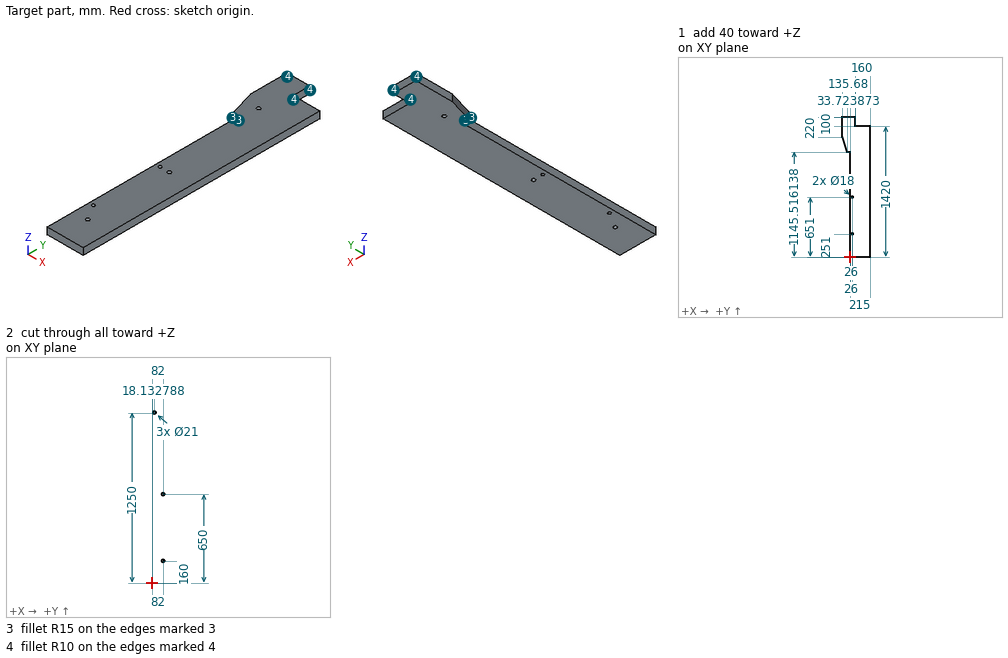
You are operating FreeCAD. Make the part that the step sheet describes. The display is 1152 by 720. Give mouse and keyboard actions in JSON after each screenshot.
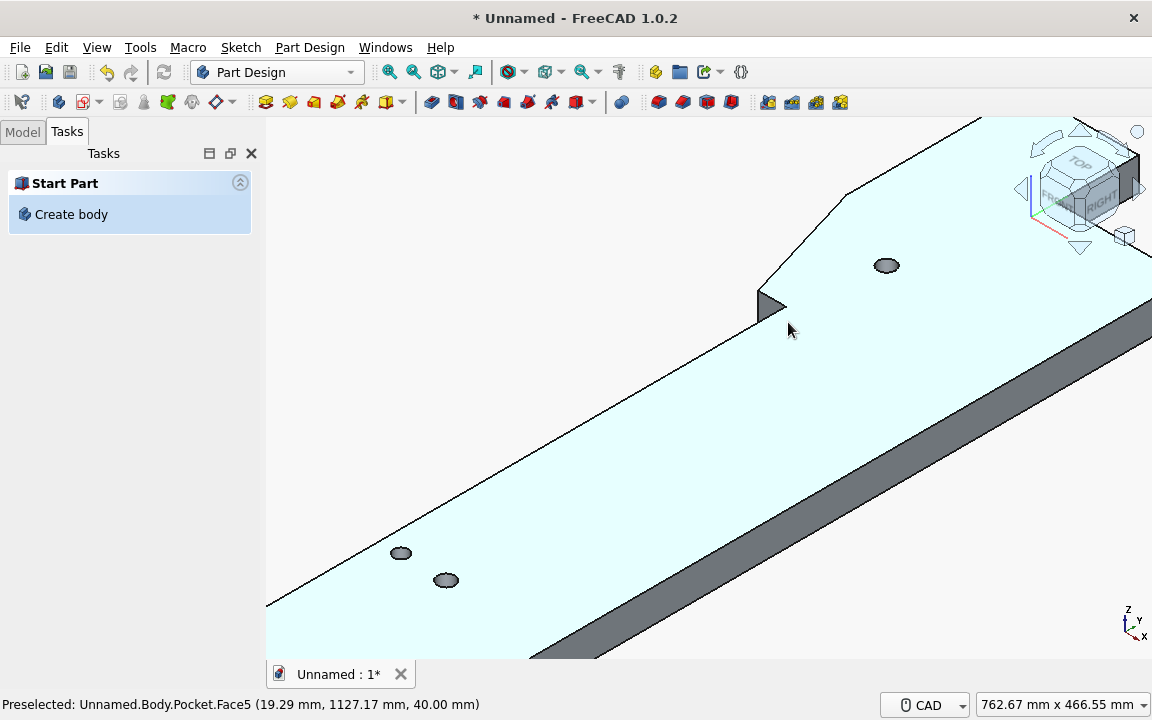
{"action": "key", "text": "v f"}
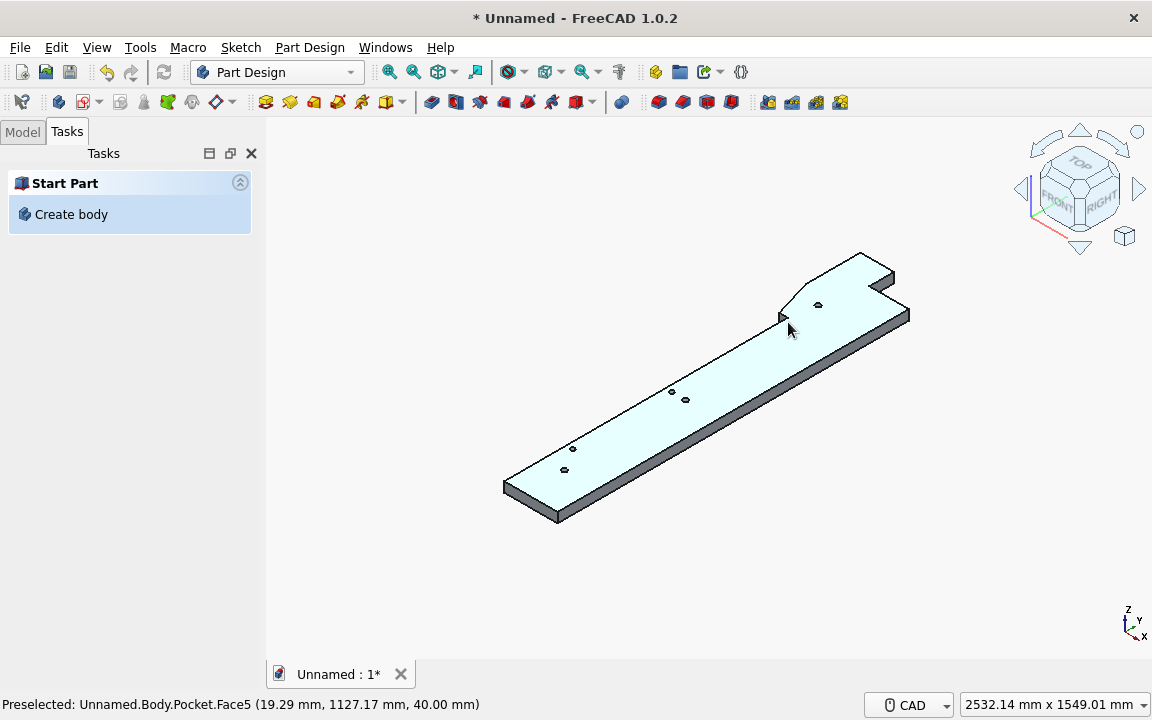
{"action": "key", "text": "2"}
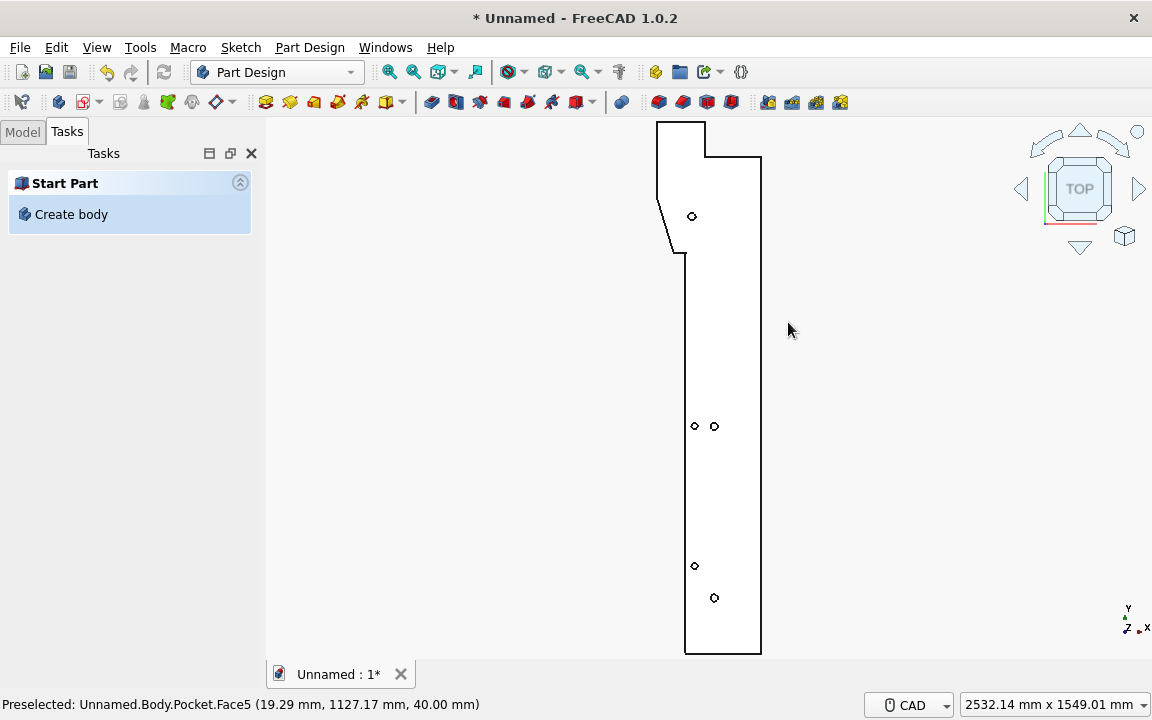
{"action": "scroll", "coordinate": [686, 252], "scroll_direction": "up", "scroll_amount": 6}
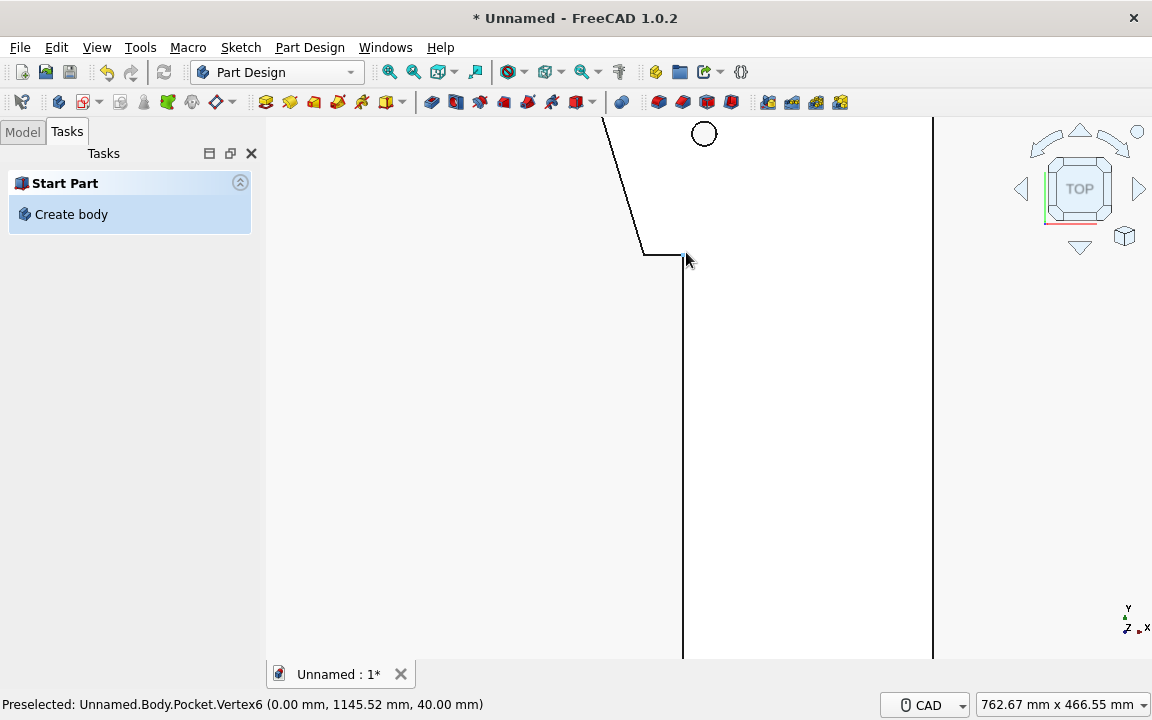
{"action": "left_click", "coordinate": [390, 72]}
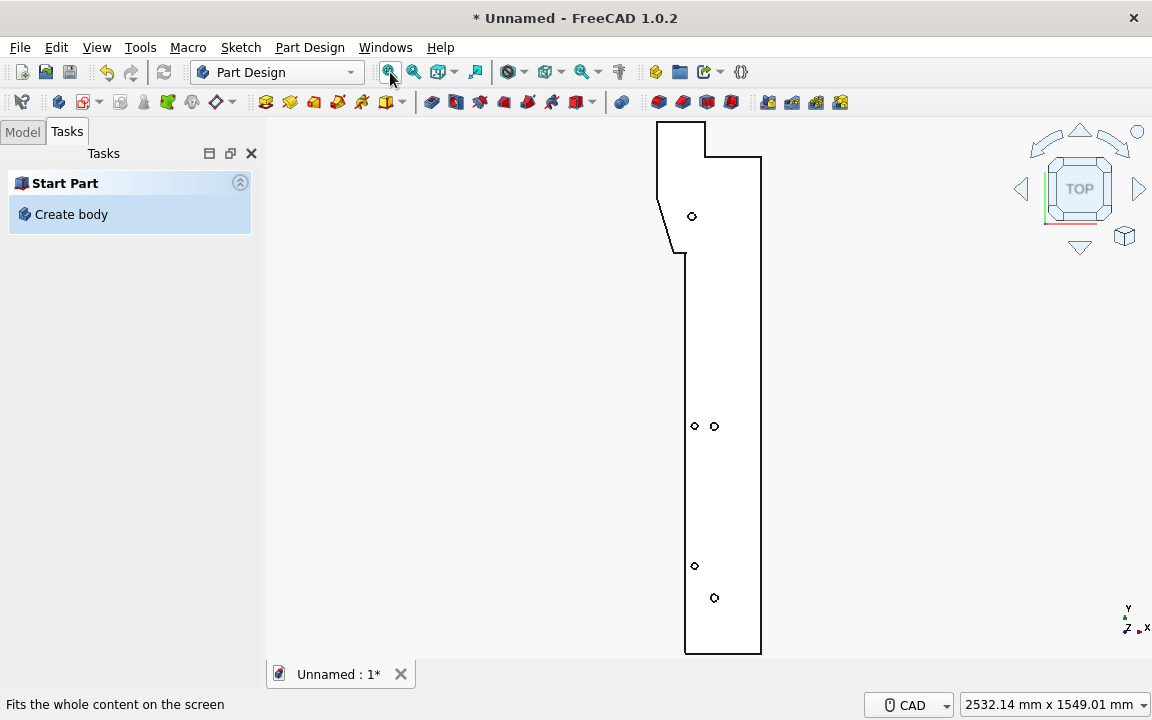
{"action": "key", "text": "1"}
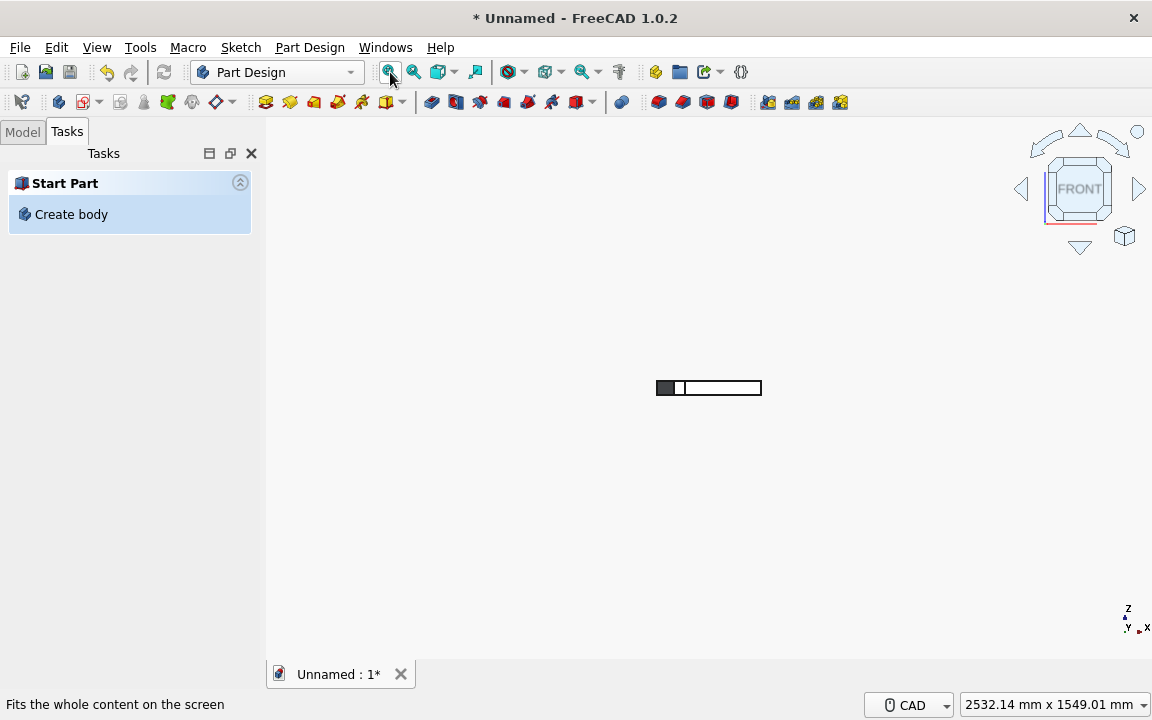
{"action": "key", "text": "v f"}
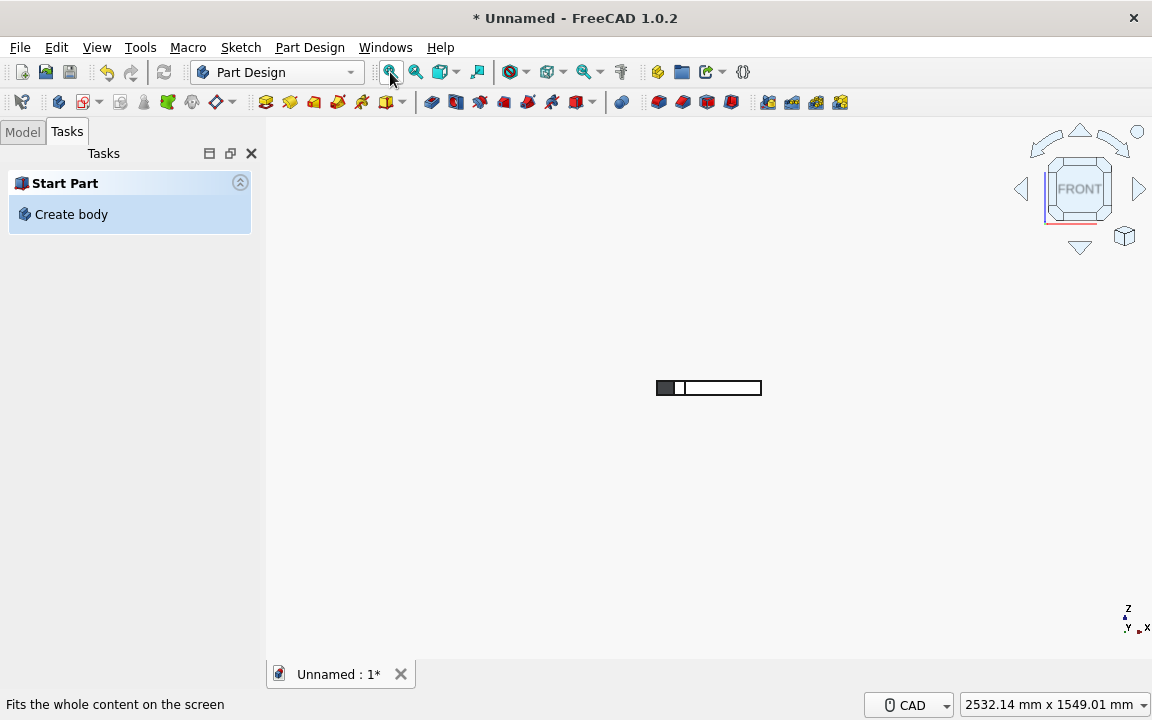
{"action": "left_click", "coordinate": [674, 387]}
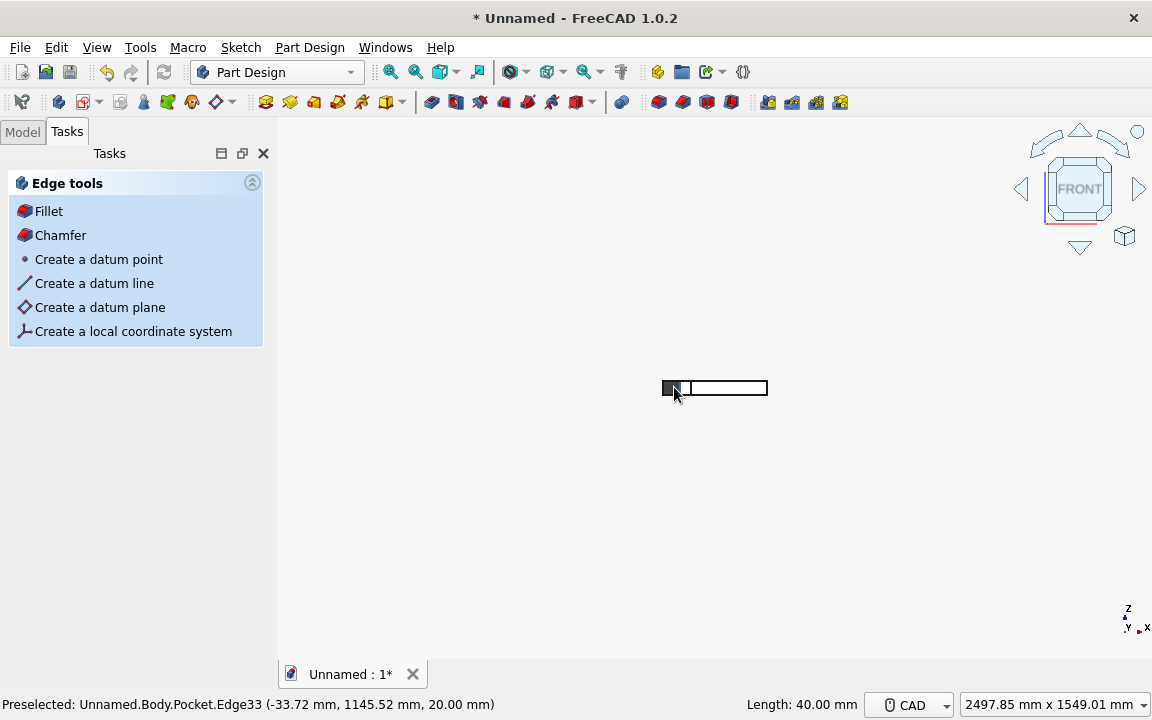
{"action": "scroll", "coordinate": [692, 387], "scroll_direction": "up", "scroll_amount": 6}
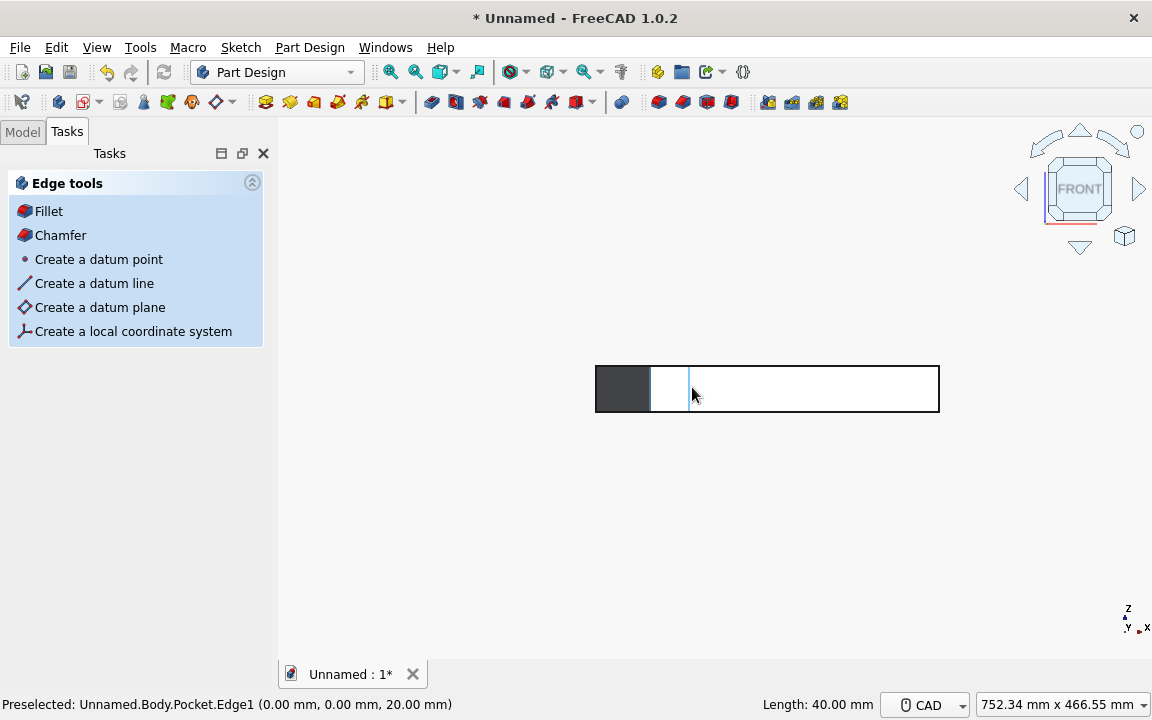
{"action": "left_click", "coordinate": [392, 72]}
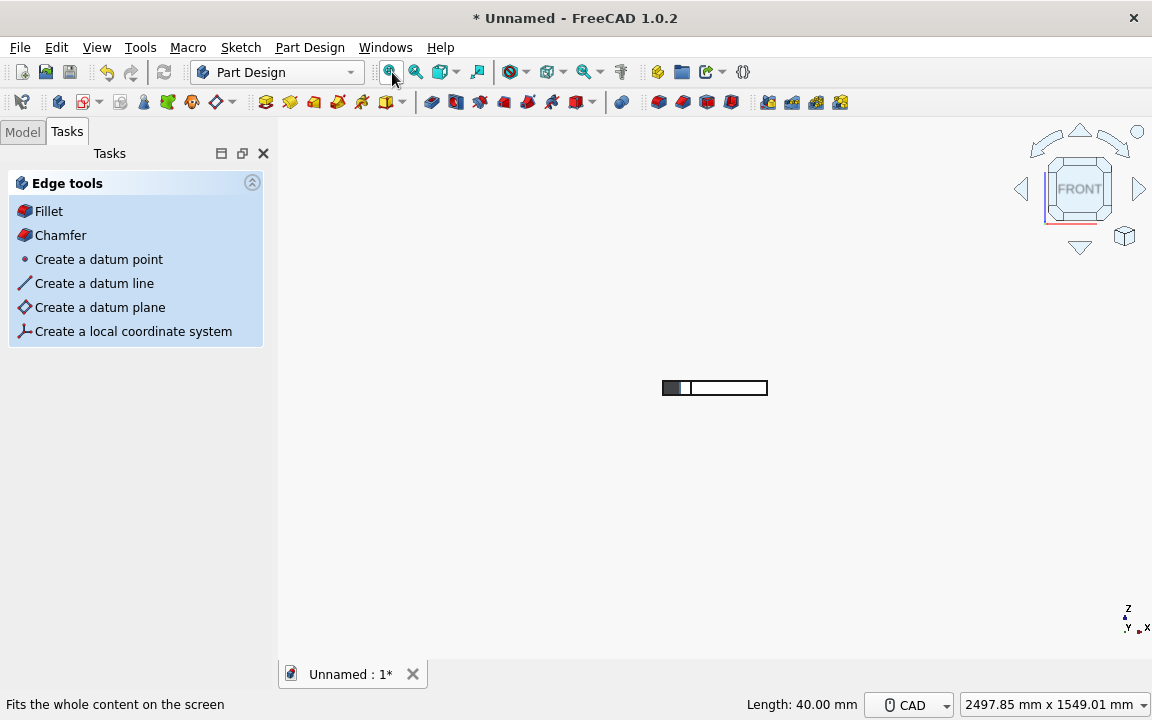
{"action": "key", "text": "3"}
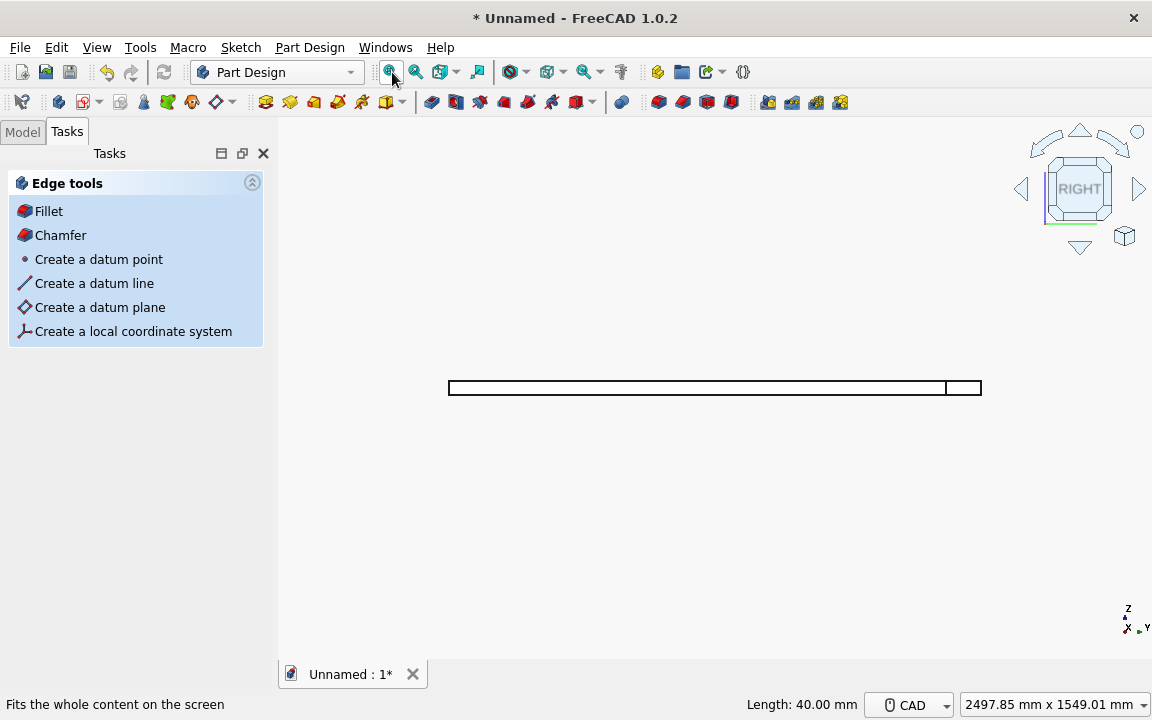
{"action": "scroll", "coordinate": [850, 387], "scroll_direction": "up", "scroll_amount": 6}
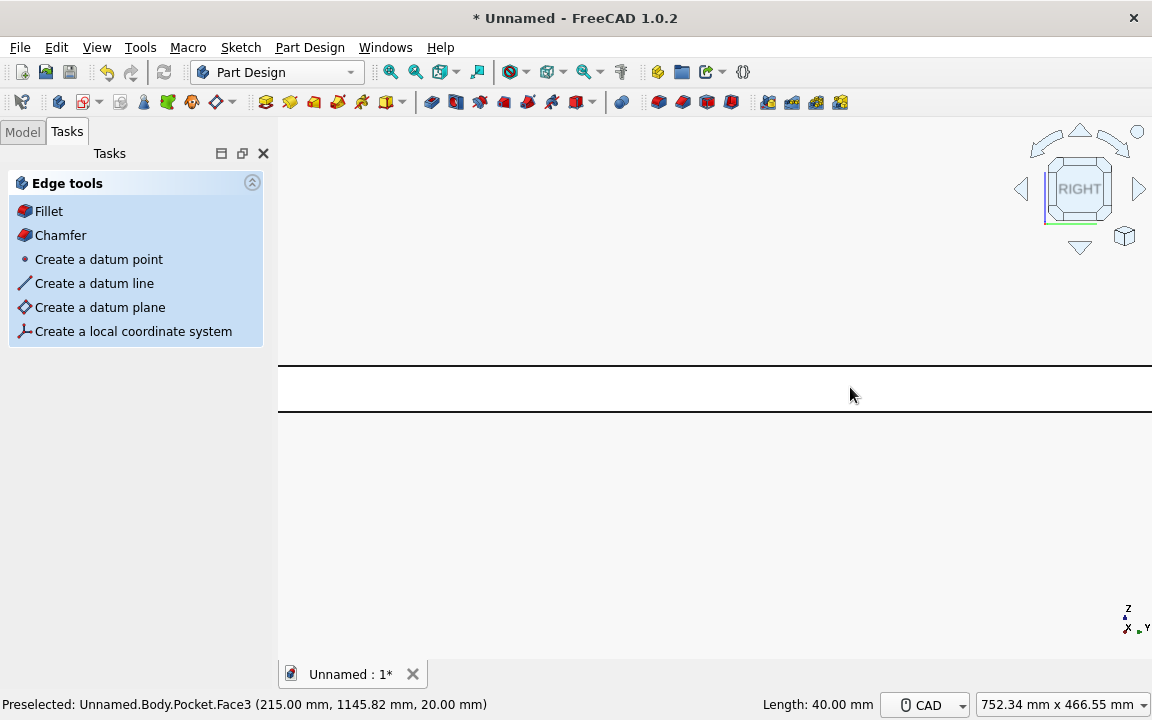
{"action": "key", "text": "v f"}